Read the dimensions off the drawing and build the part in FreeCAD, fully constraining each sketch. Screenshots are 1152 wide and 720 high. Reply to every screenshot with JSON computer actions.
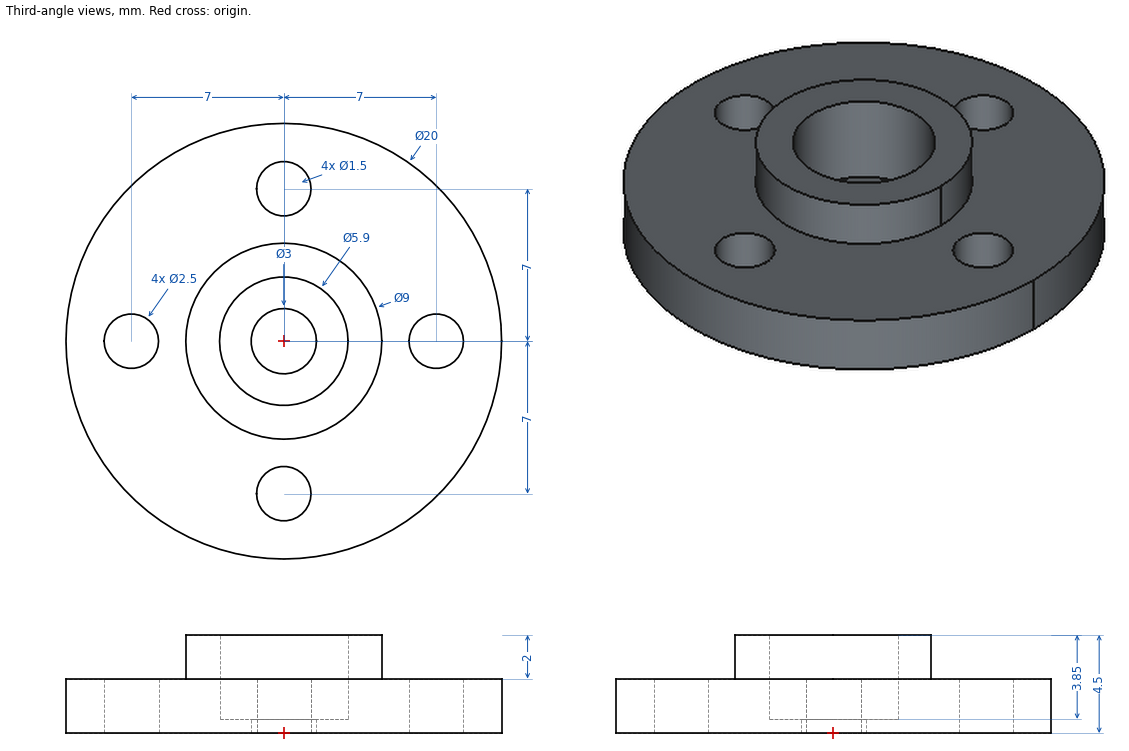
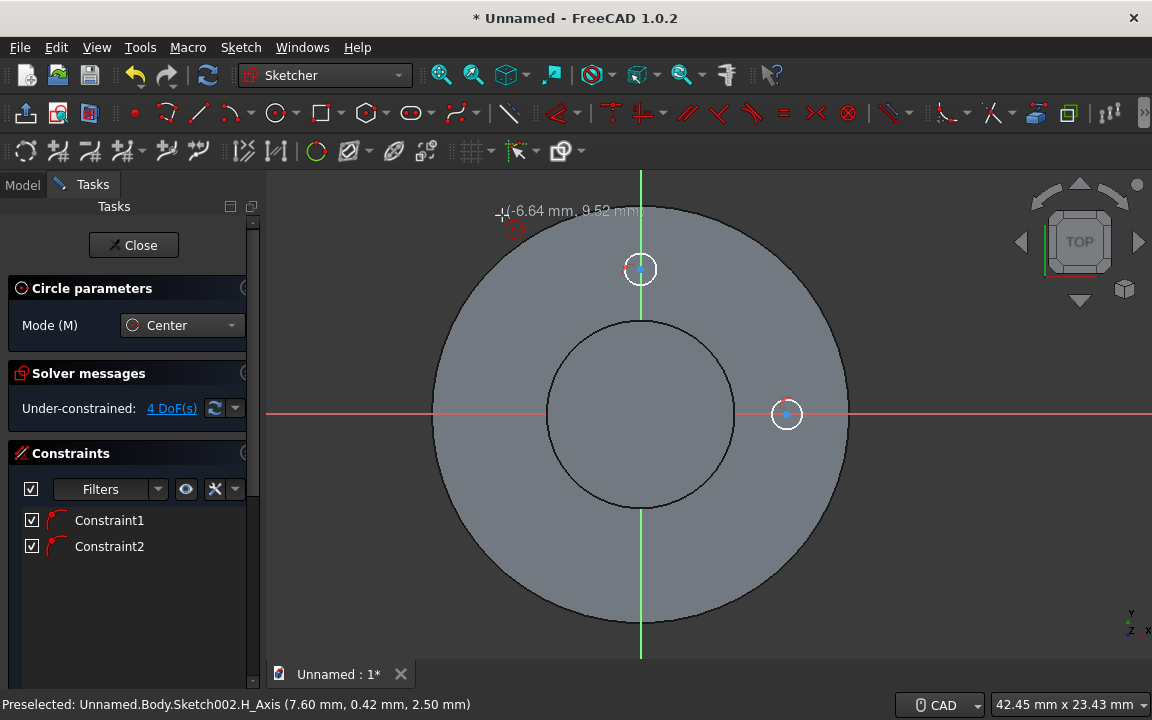
{"action": "scroll", "coordinate": [641, 561], "scroll_direction": "up", "scroll_amount": 2}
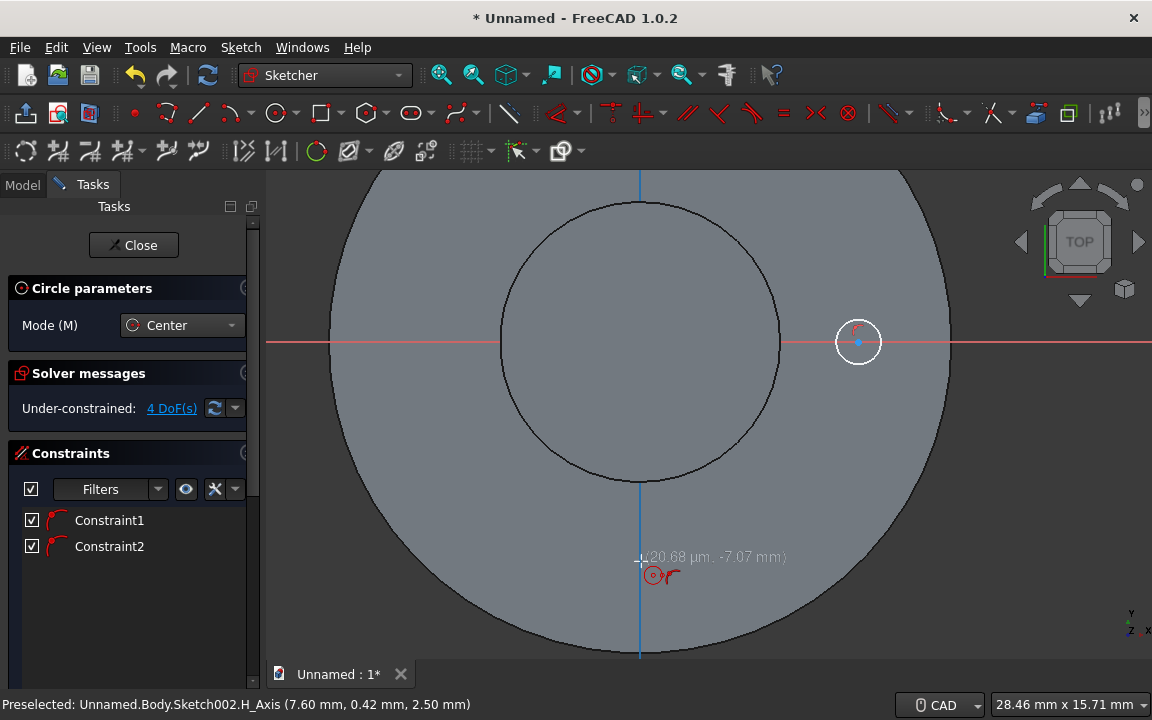
{"action": "left_click", "coordinate": [640, 560]}
{"action": "left_click", "coordinate": [657, 543]}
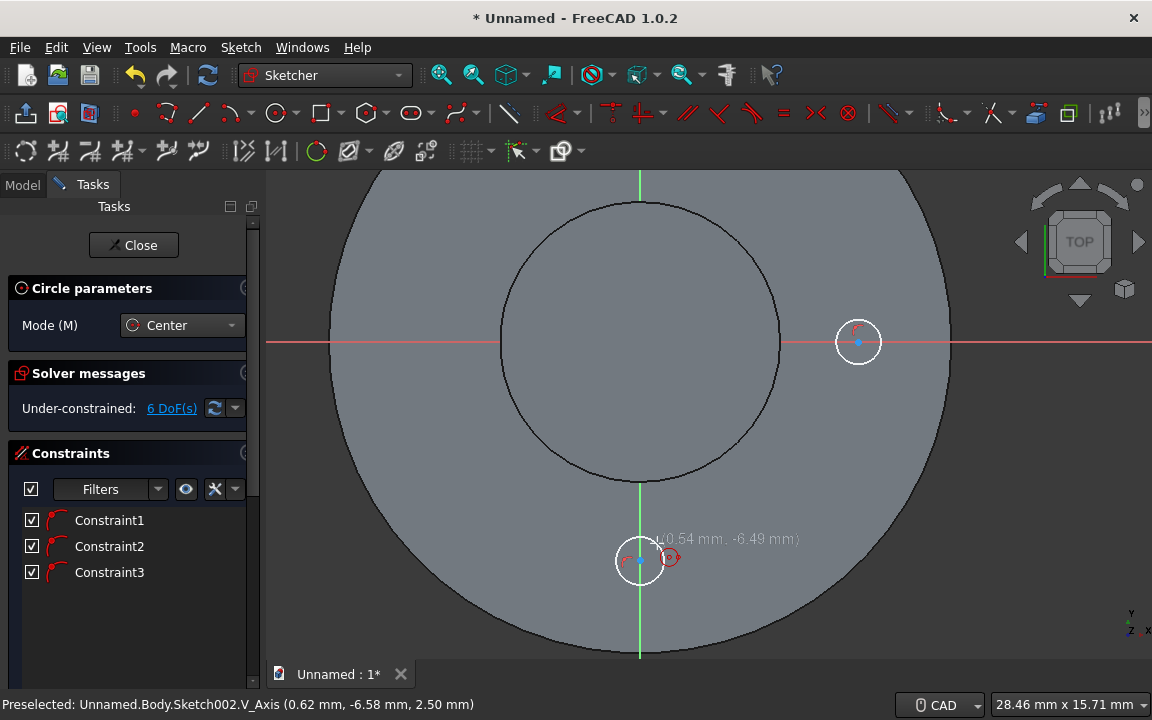
{"action": "left_click", "coordinate": [422, 342]}
{"action": "left_click", "coordinate": [439, 326]}
{"action": "key", "text": "Escape"}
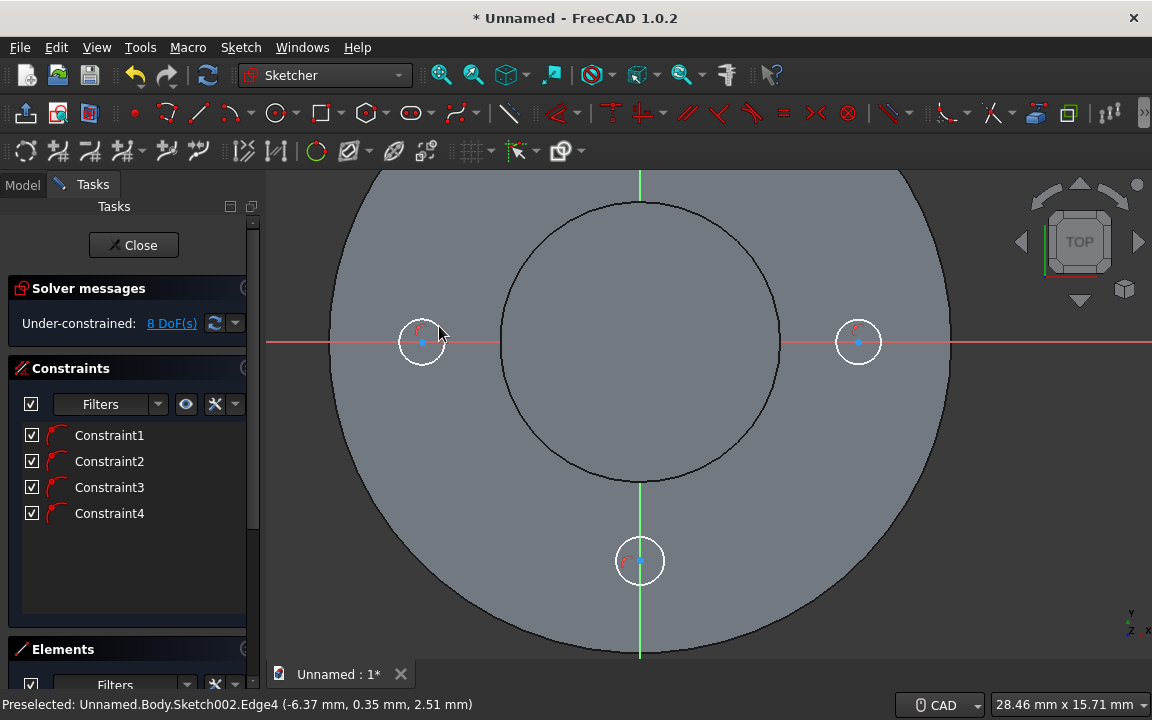
{"action": "scroll", "coordinate": [641, 562], "scroll_direction": "down", "scroll_amount": 2}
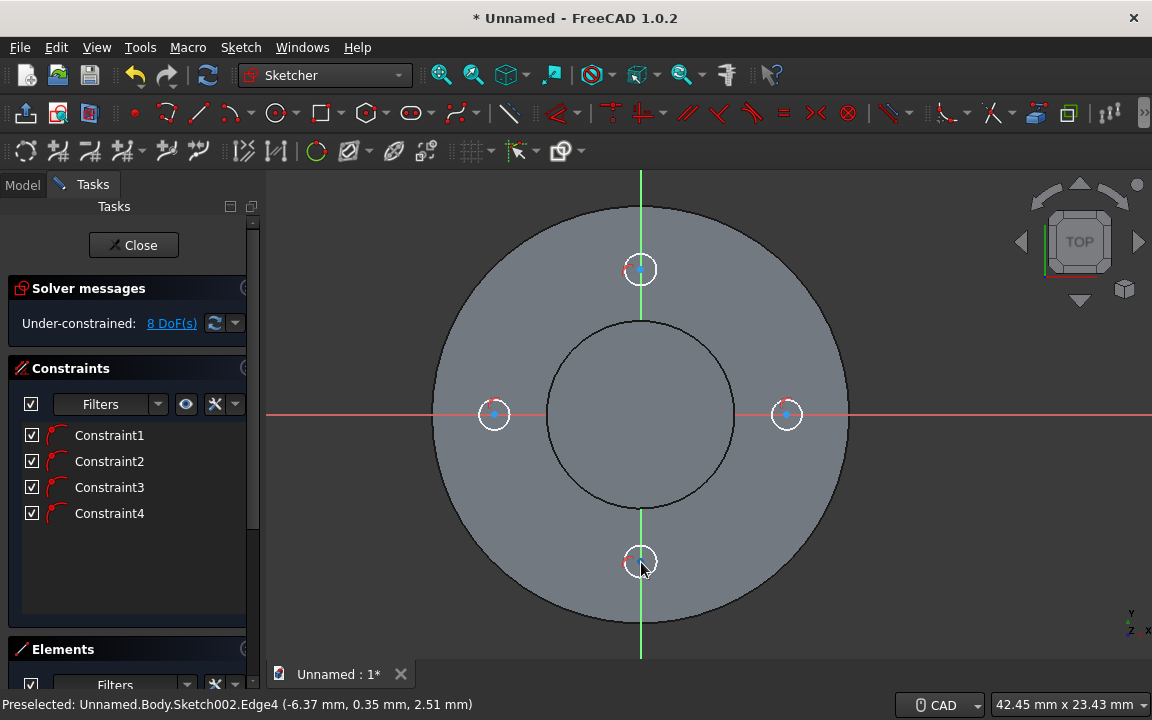
{"action": "scroll", "coordinate": [652, 258], "scroll_direction": "up", "scroll_amount": 2}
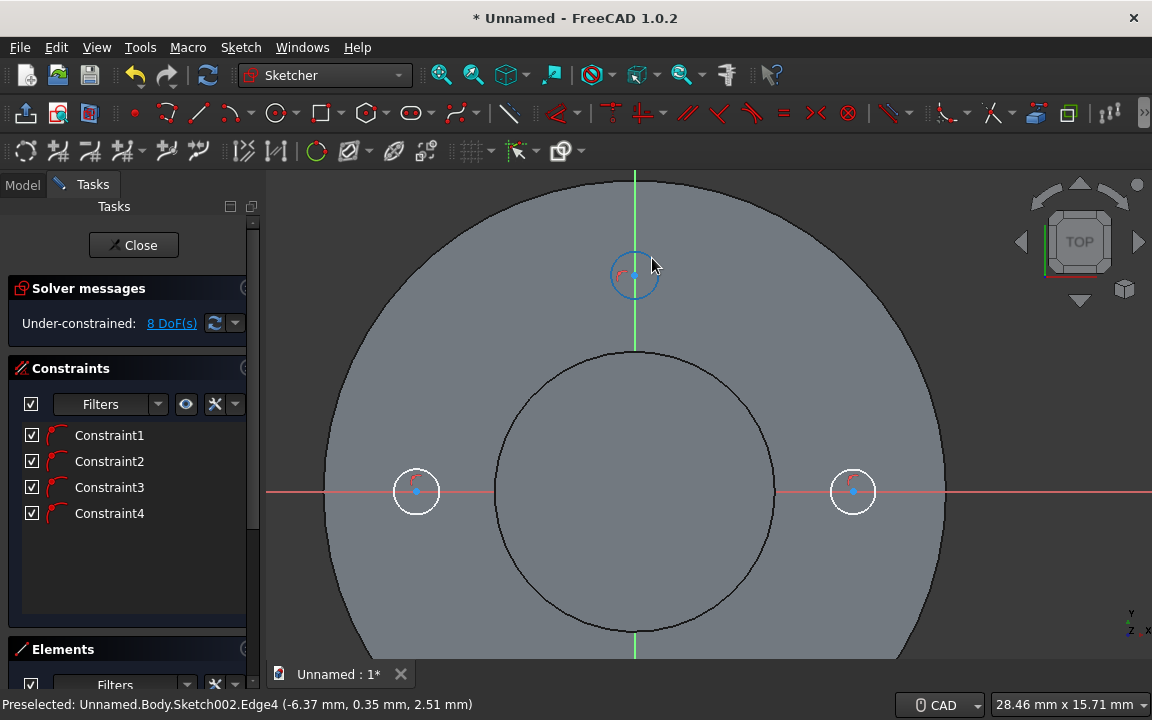
{"action": "left_click", "coordinate": [651, 259]}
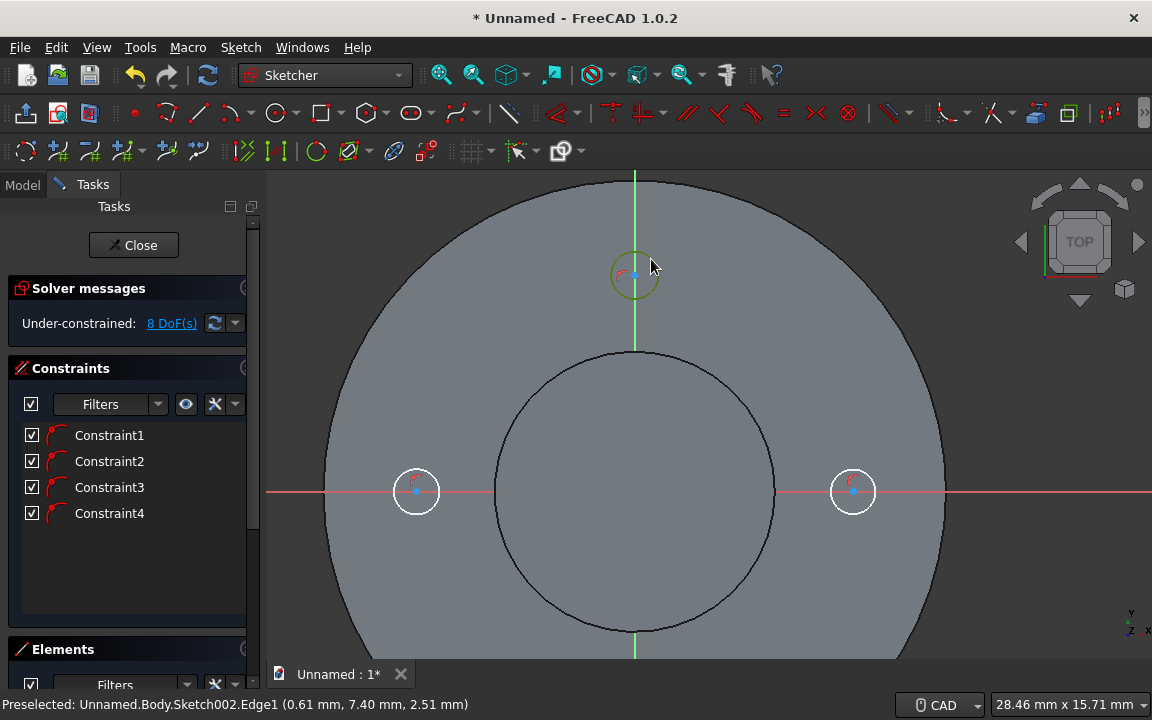
{"action": "left_click", "coordinate": [869, 476]}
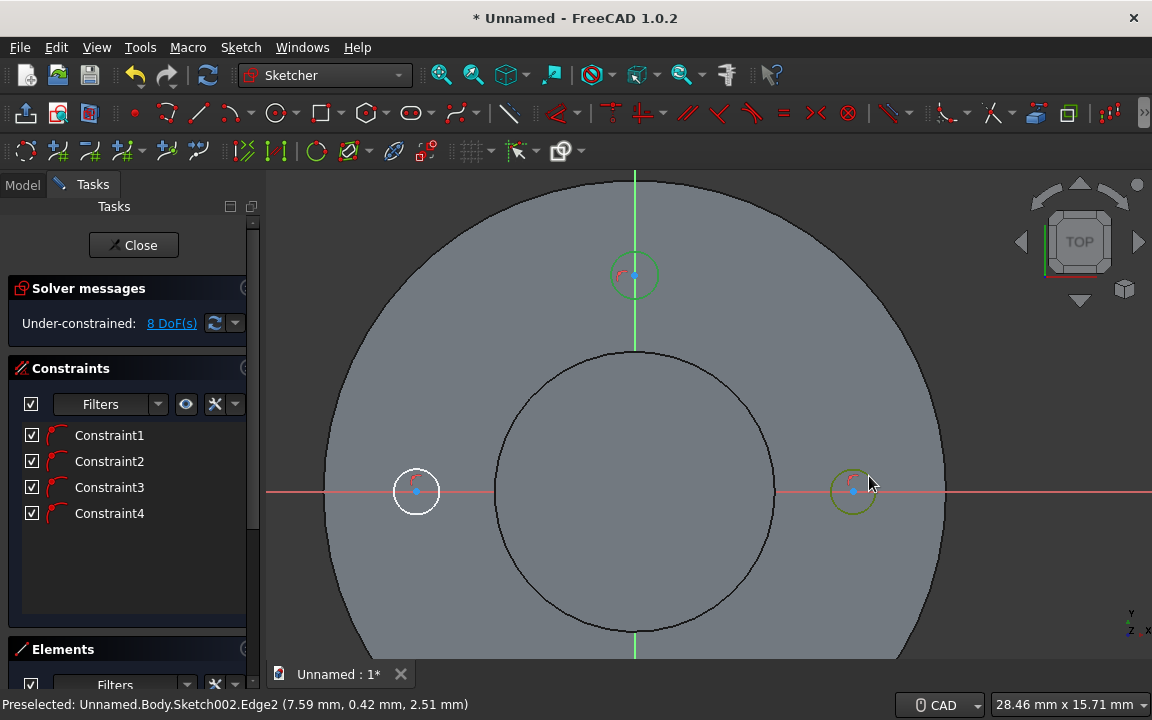
{"action": "scroll", "coordinate": [652, 257], "scroll_direction": "down", "scroll_amount": 2}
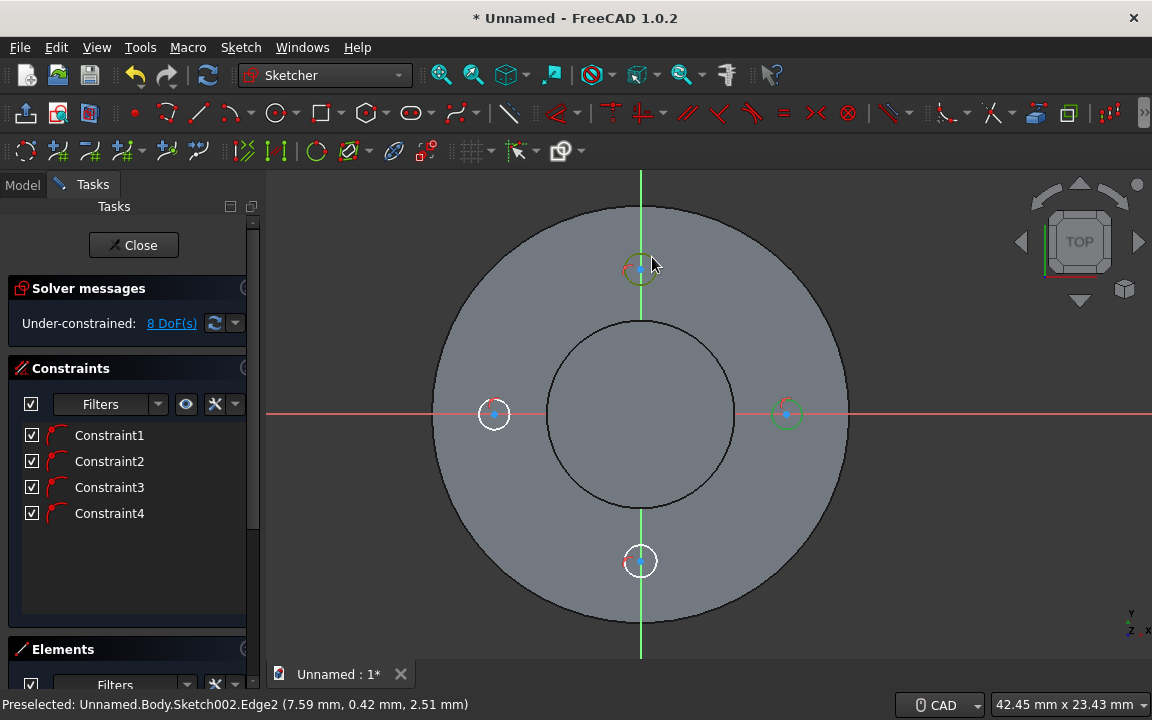
{"action": "left_click", "coordinate": [652, 550]}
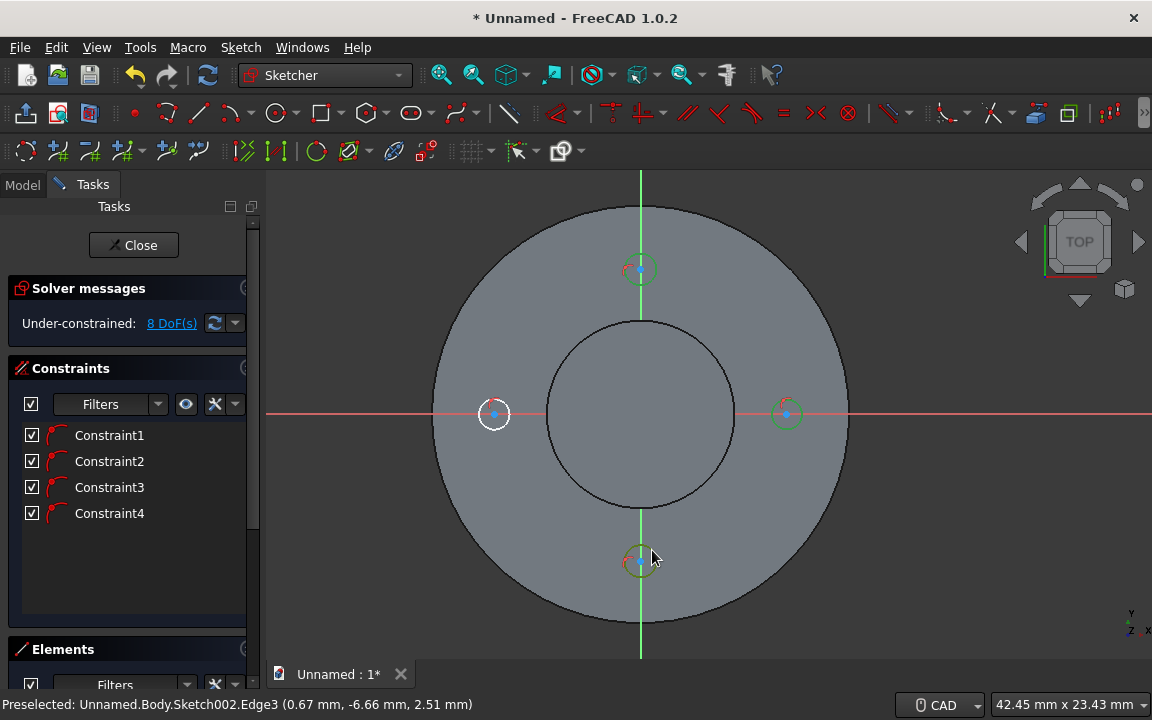
{"action": "scroll", "coordinate": [505, 404], "scroll_direction": "up", "scroll_amount": 2}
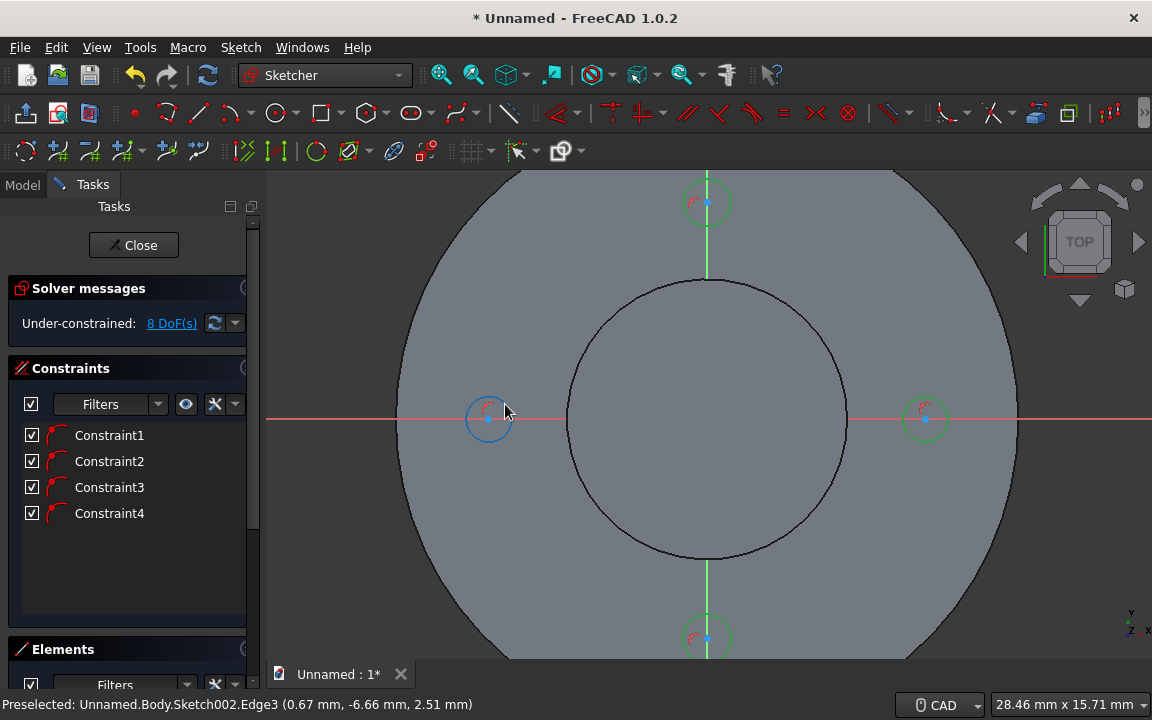
{"action": "left_click", "coordinate": [505, 403]}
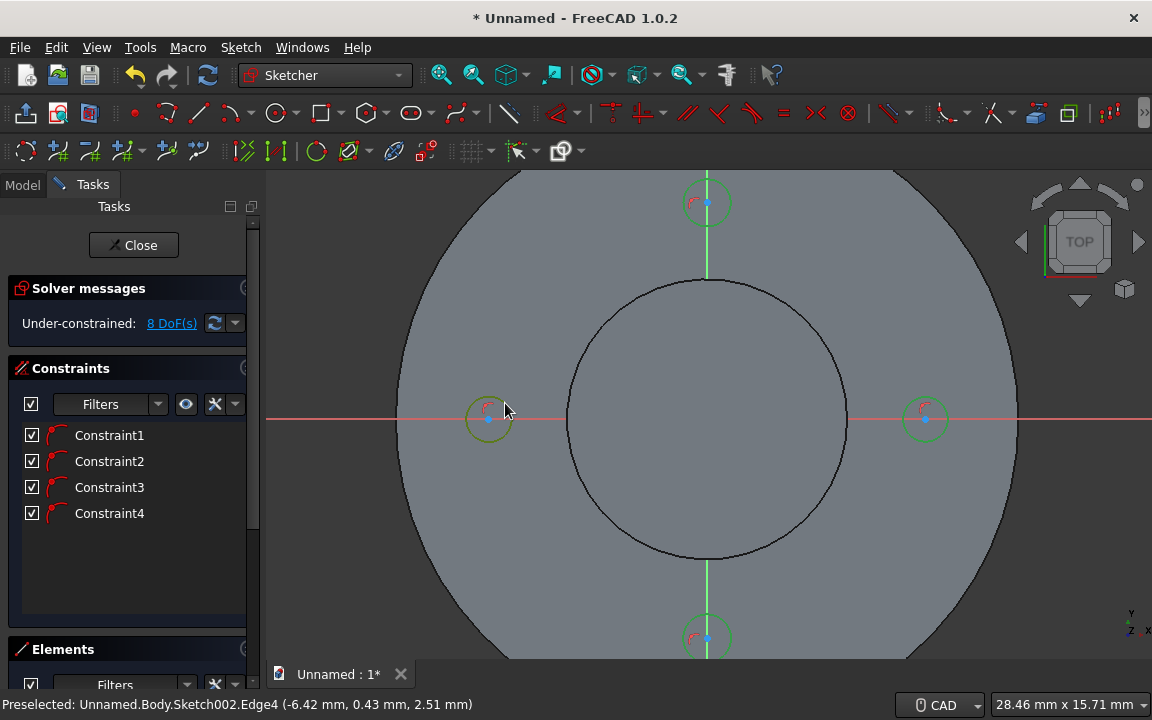
{"action": "left_click", "coordinate": [784, 114]}